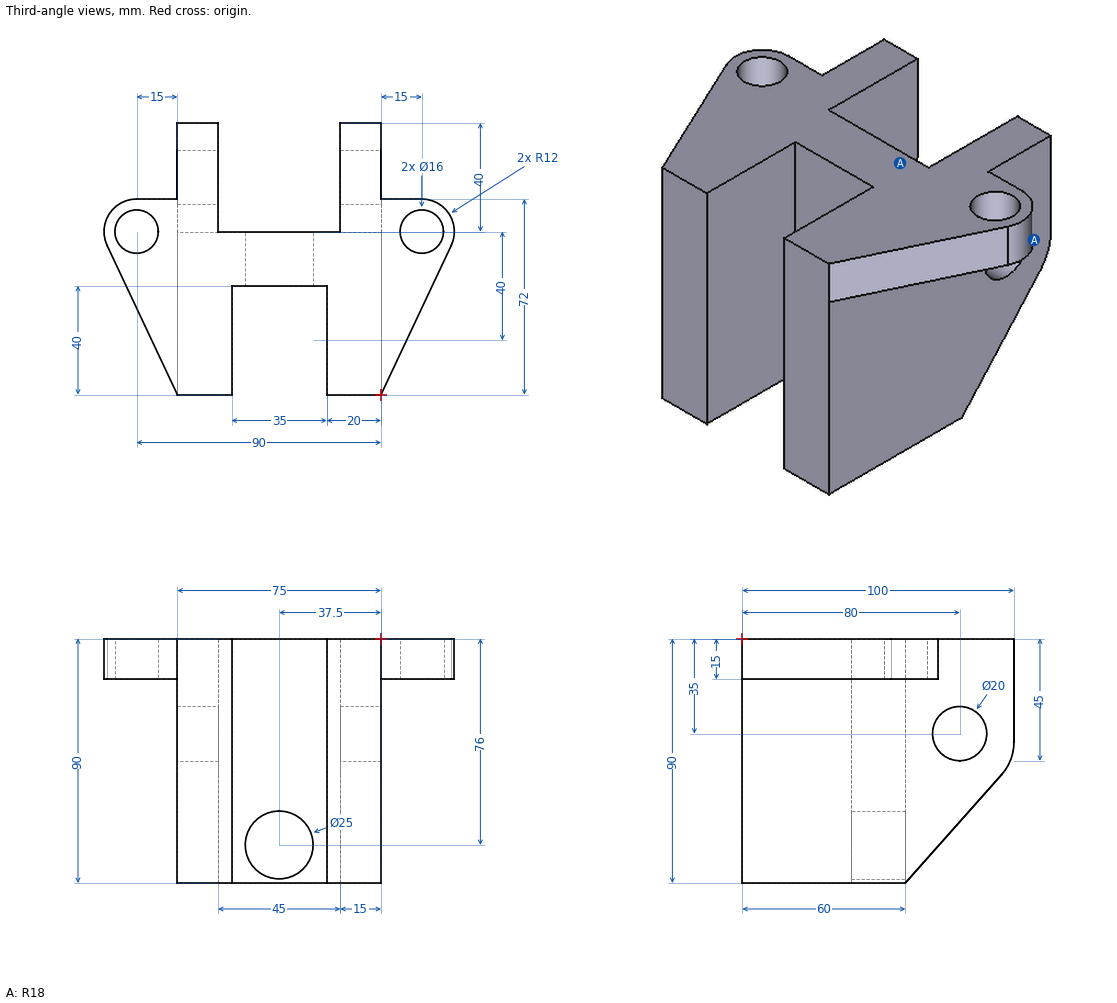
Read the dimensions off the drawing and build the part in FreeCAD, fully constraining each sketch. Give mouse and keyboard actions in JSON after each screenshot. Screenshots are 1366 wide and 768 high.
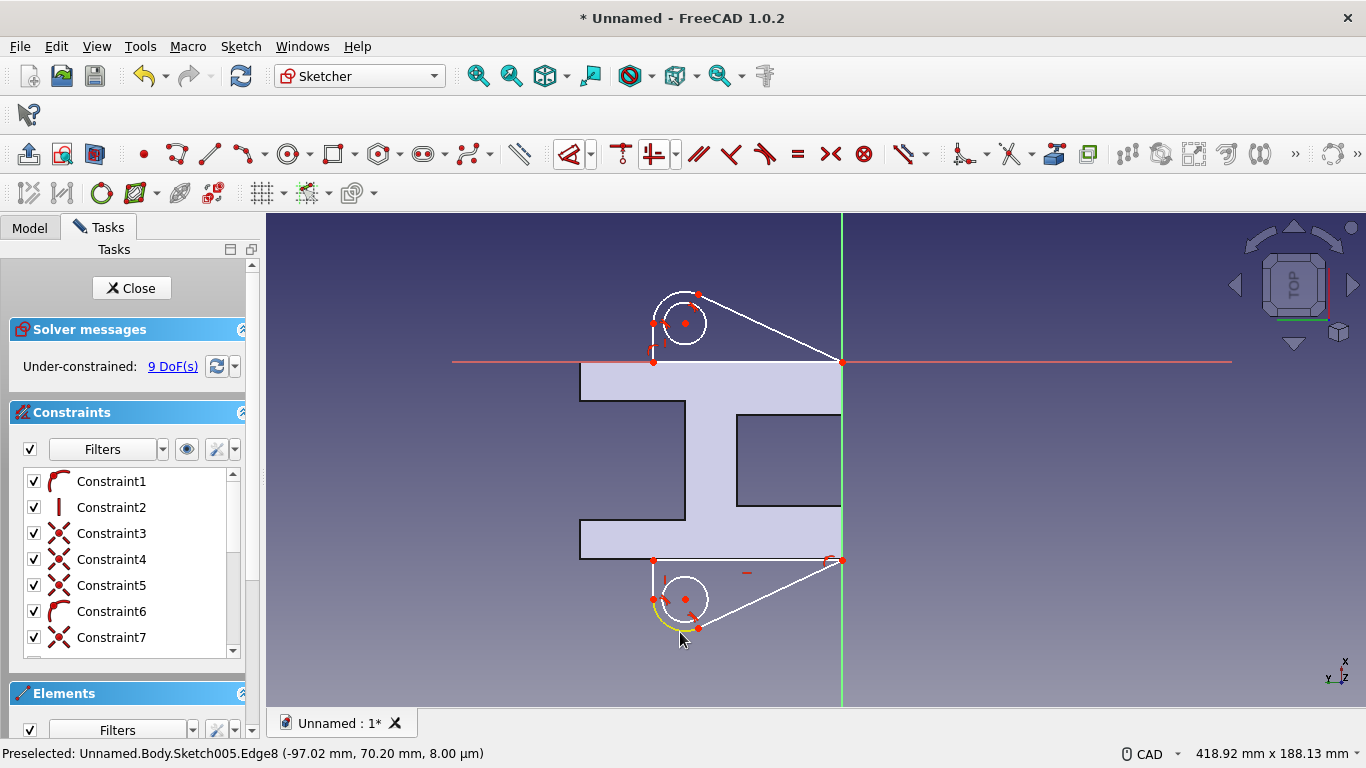
{"action": "scroll", "coordinate": [680, 292], "scroll_direction": "up", "scroll_amount": 2}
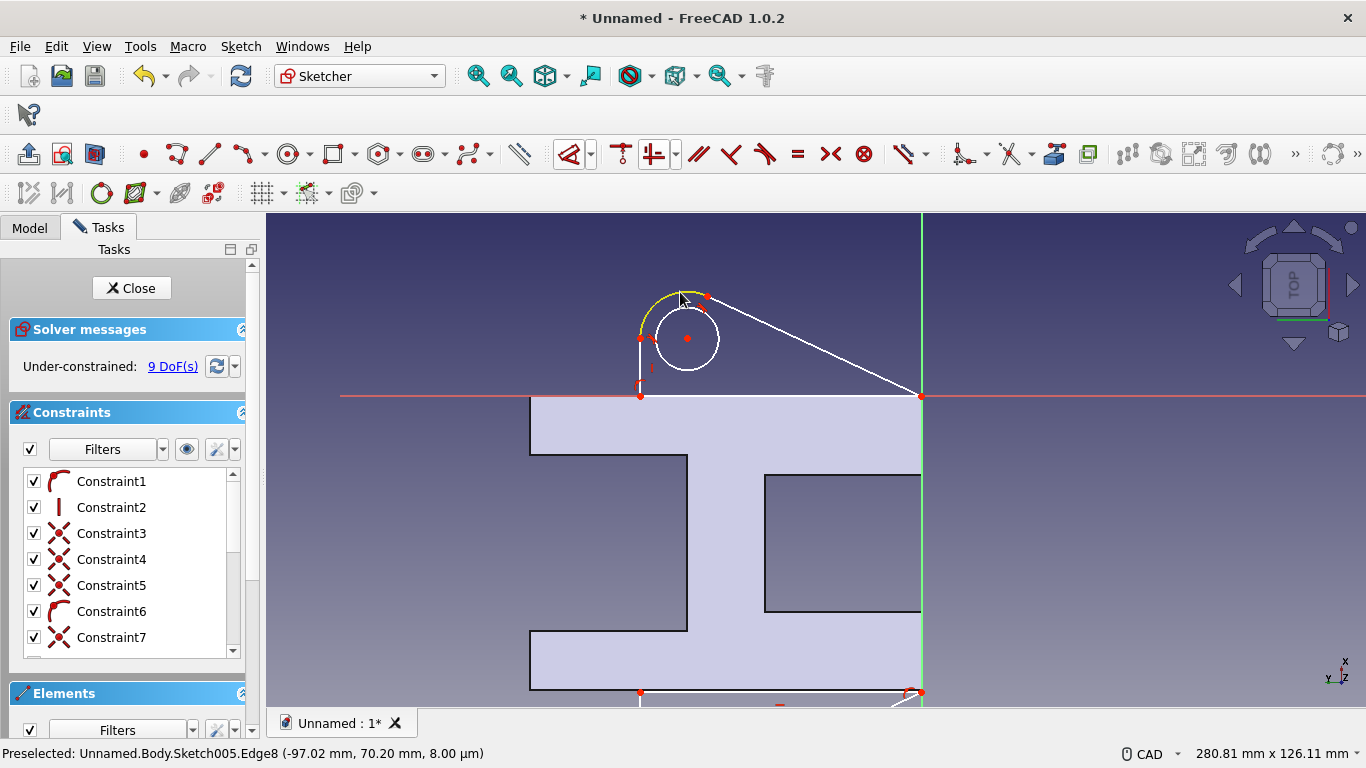
{"action": "left_click", "coordinate": [680, 292]}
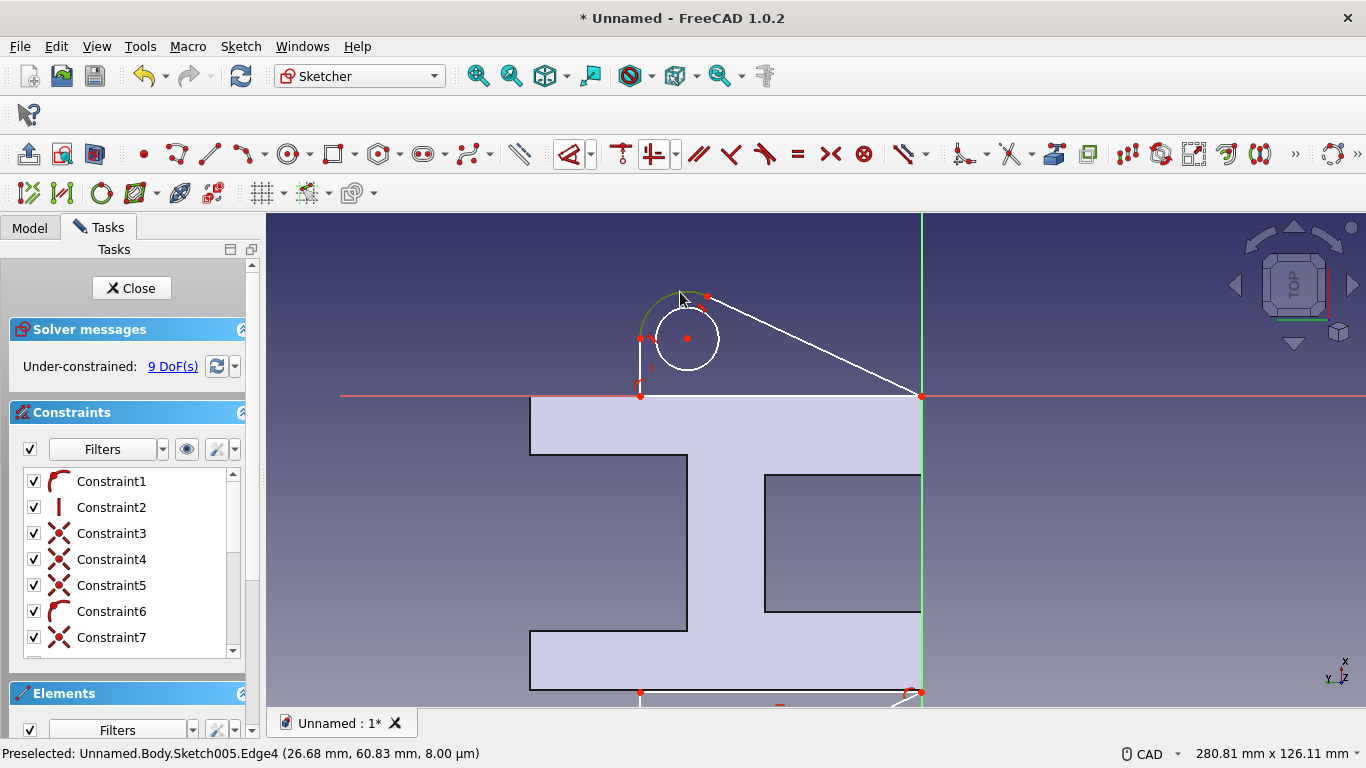
{"action": "scroll", "coordinate": [680, 291], "scroll_direction": "down", "scroll_amount": 2}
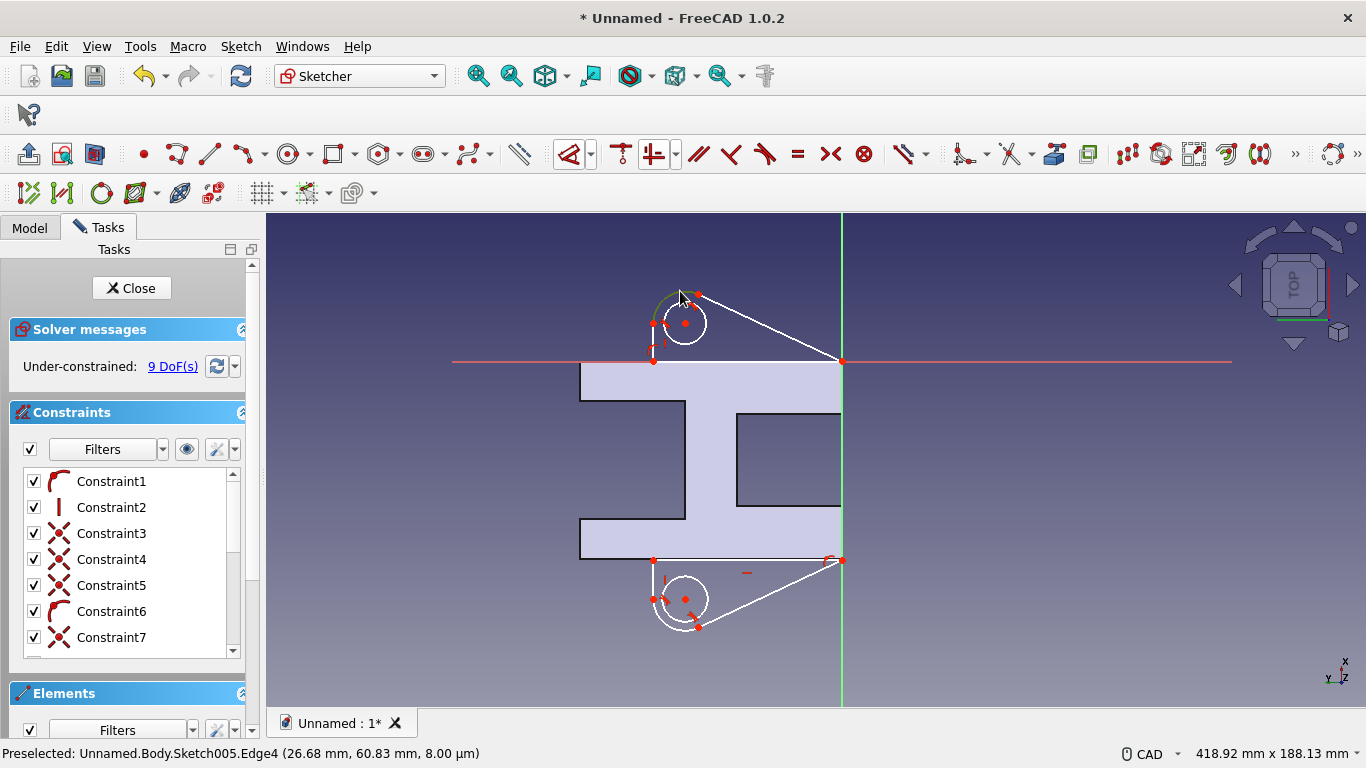
{"action": "scroll", "coordinate": [659, 617], "scroll_direction": "up", "scroll_amount": 3}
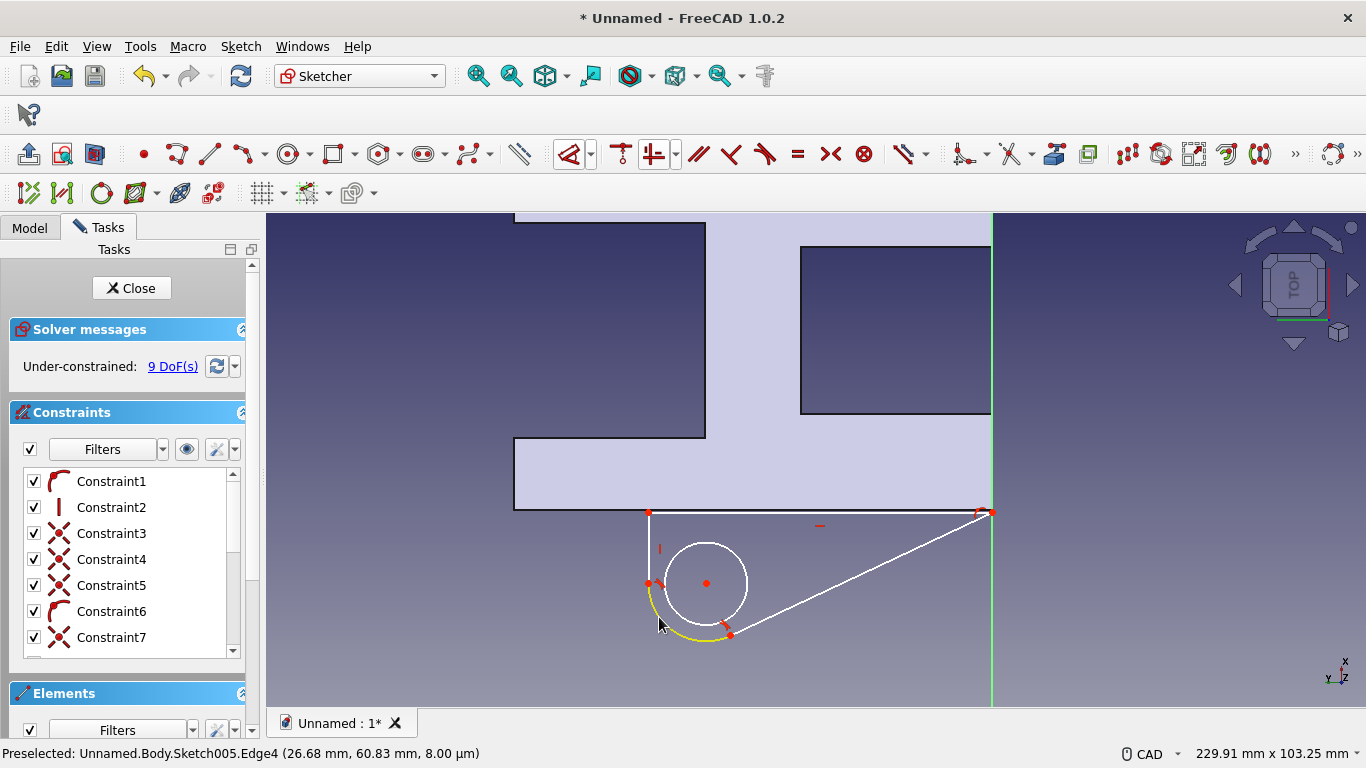
{"action": "left_click", "coordinate": [659, 616]}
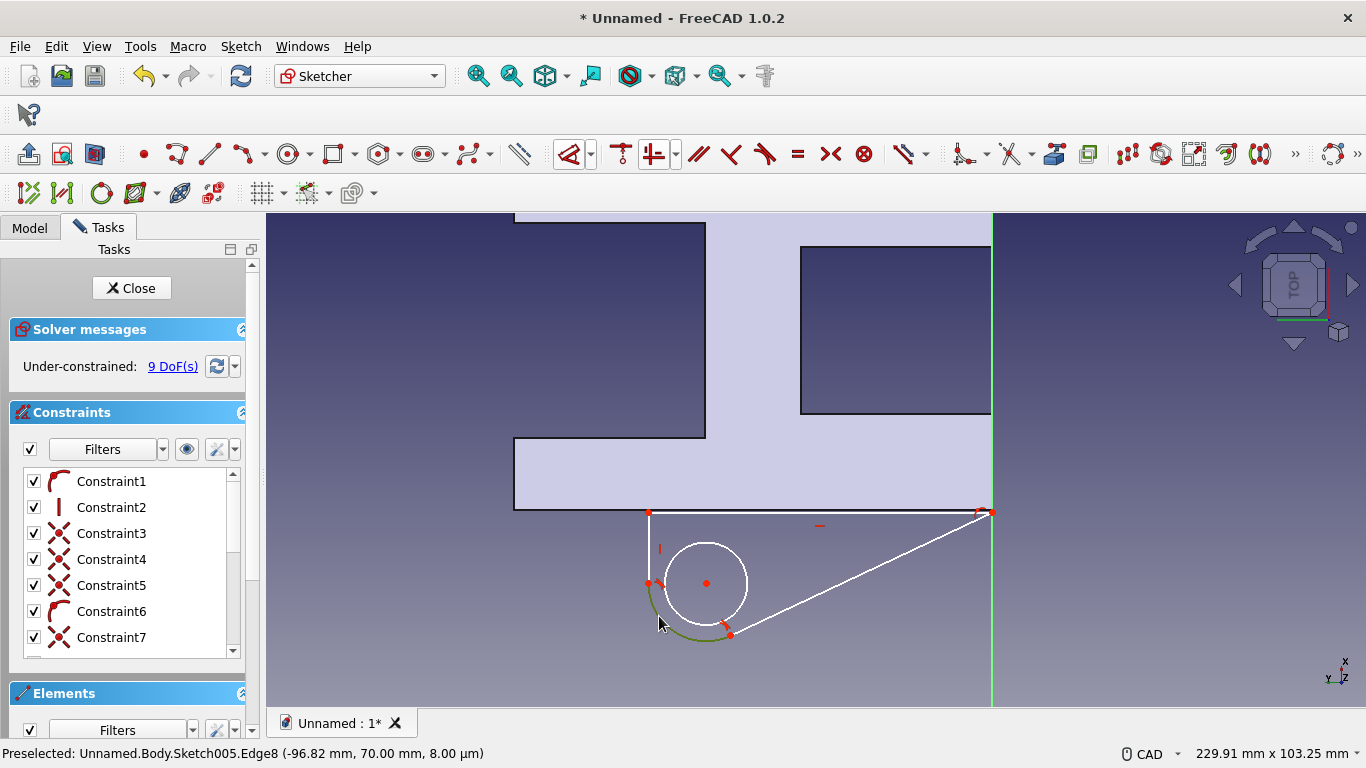
{"action": "left_click", "coordinate": [798, 154]}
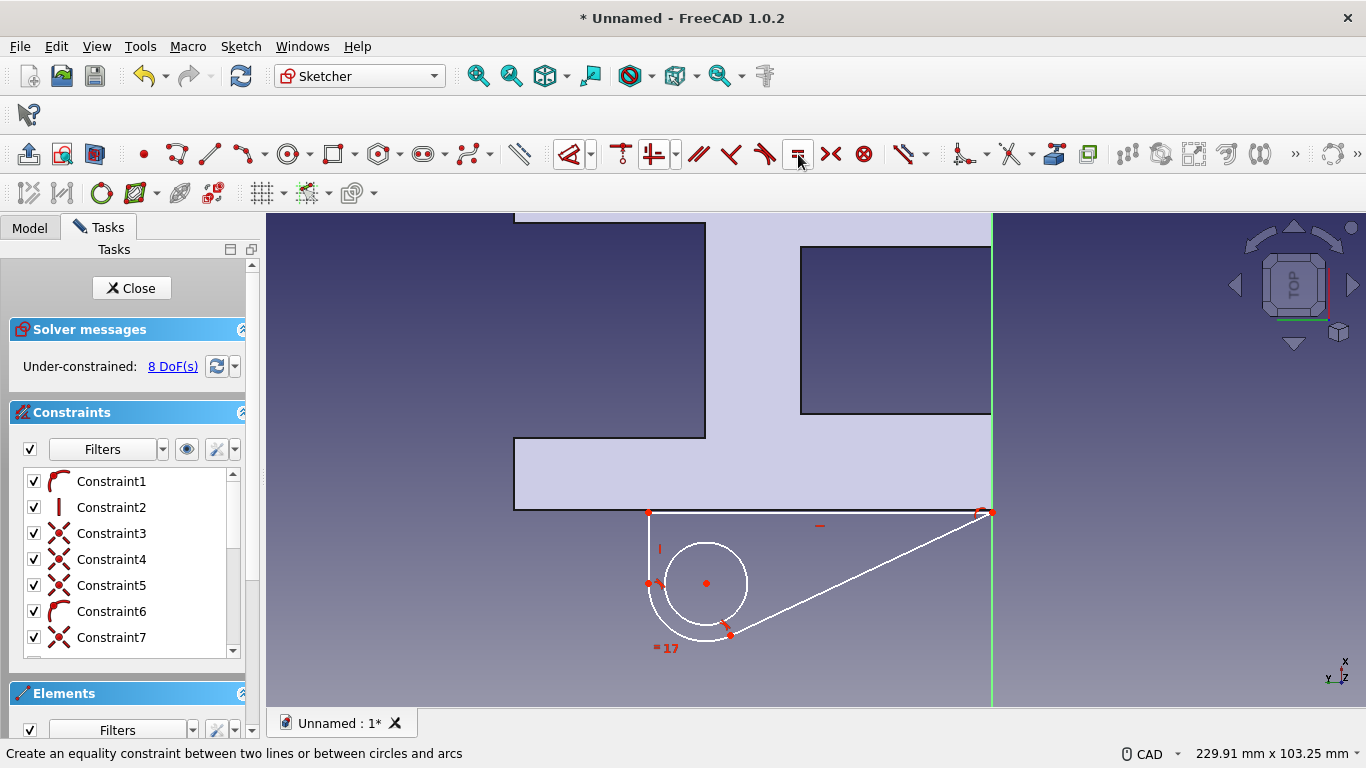
{"action": "scroll", "coordinate": [659, 617], "scroll_direction": "down", "scroll_amount": 3}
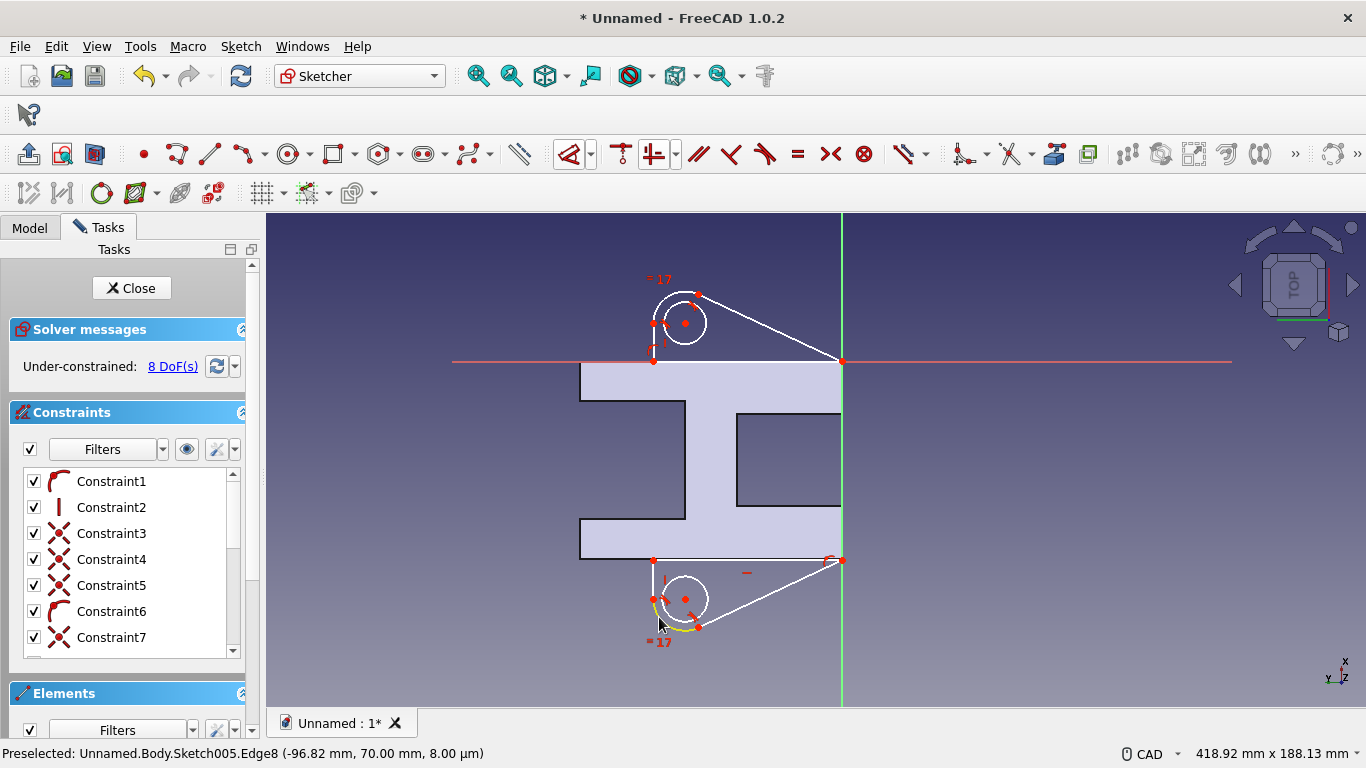
{"action": "left_click", "coordinate": [700, 308]}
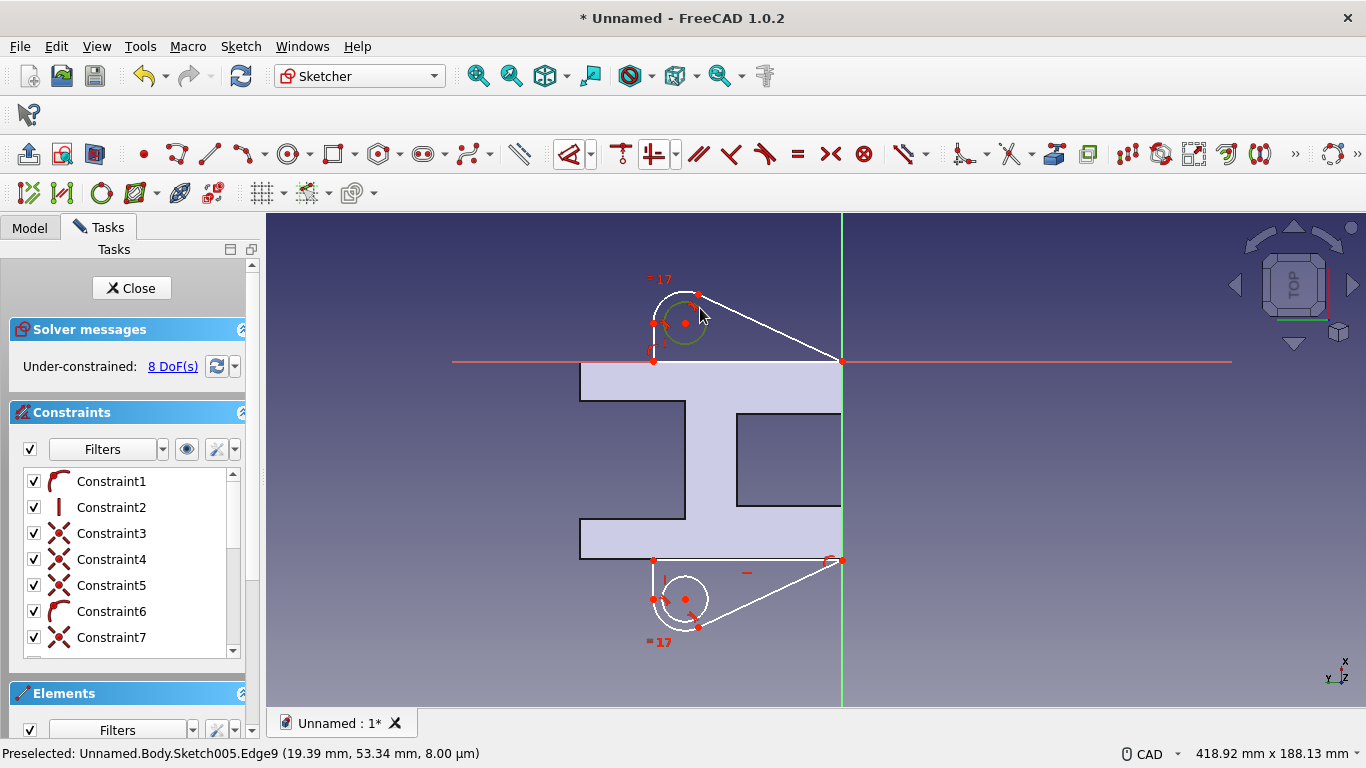
{"action": "left_click", "coordinate": [701, 583]}